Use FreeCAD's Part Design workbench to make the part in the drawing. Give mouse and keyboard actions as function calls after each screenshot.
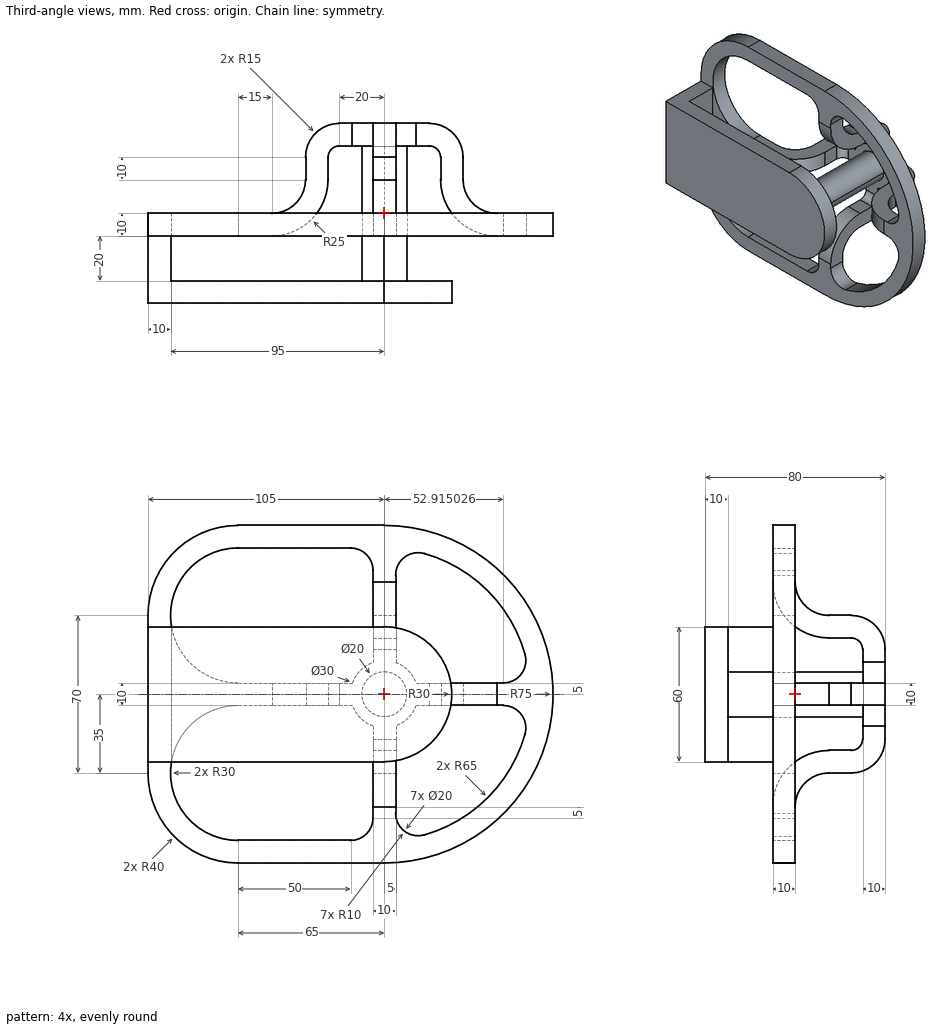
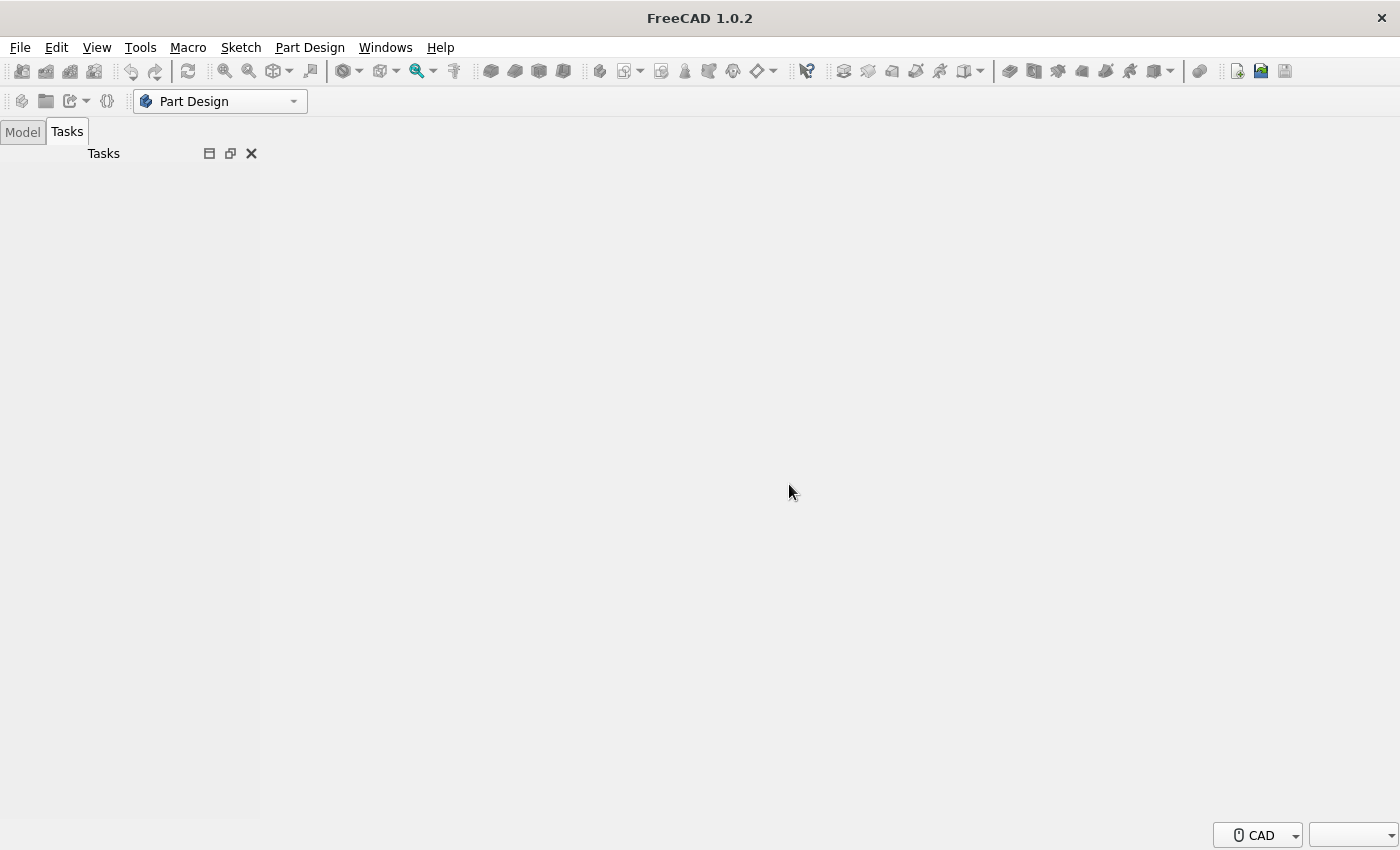
click(1238, 72)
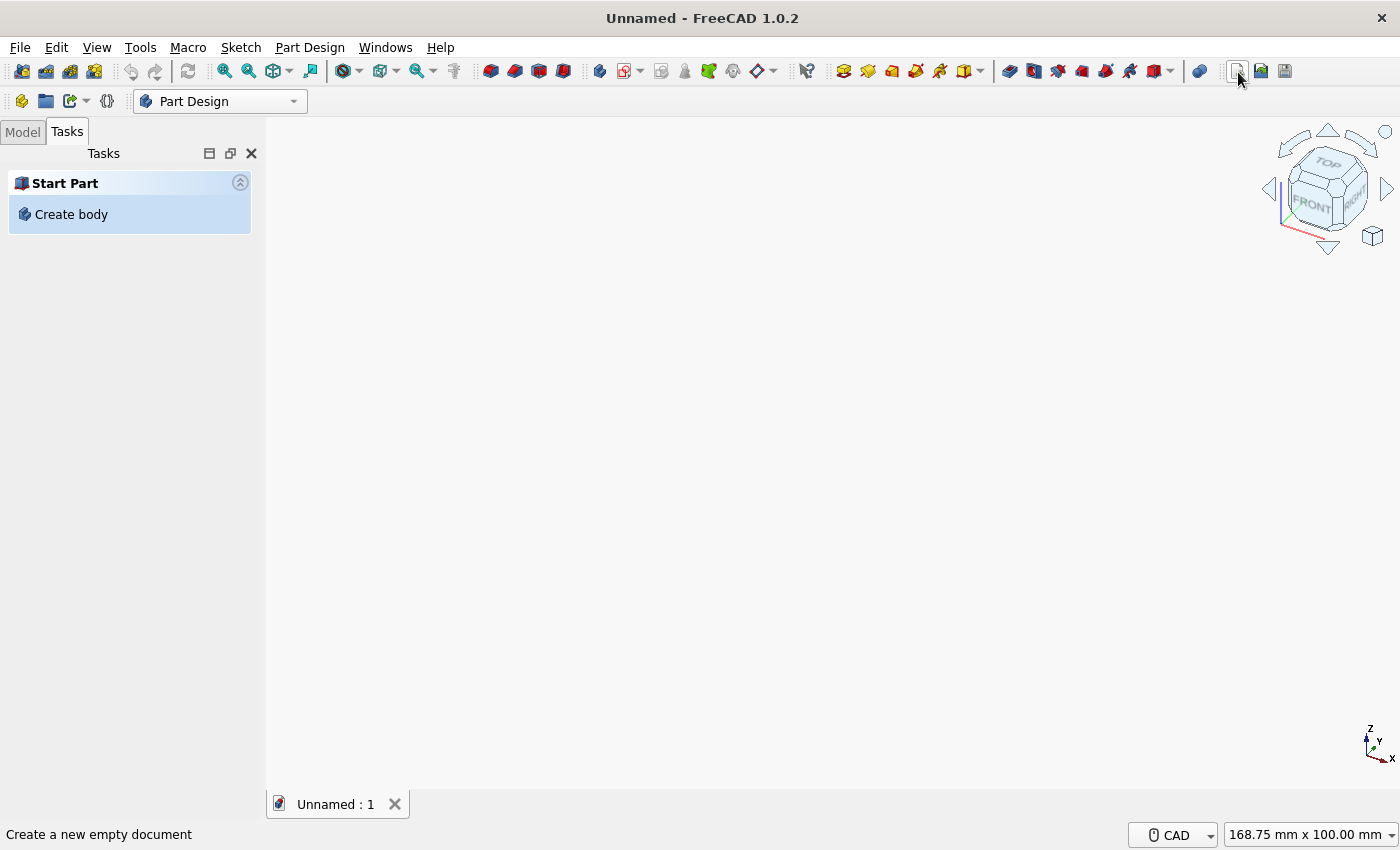
click(624, 72)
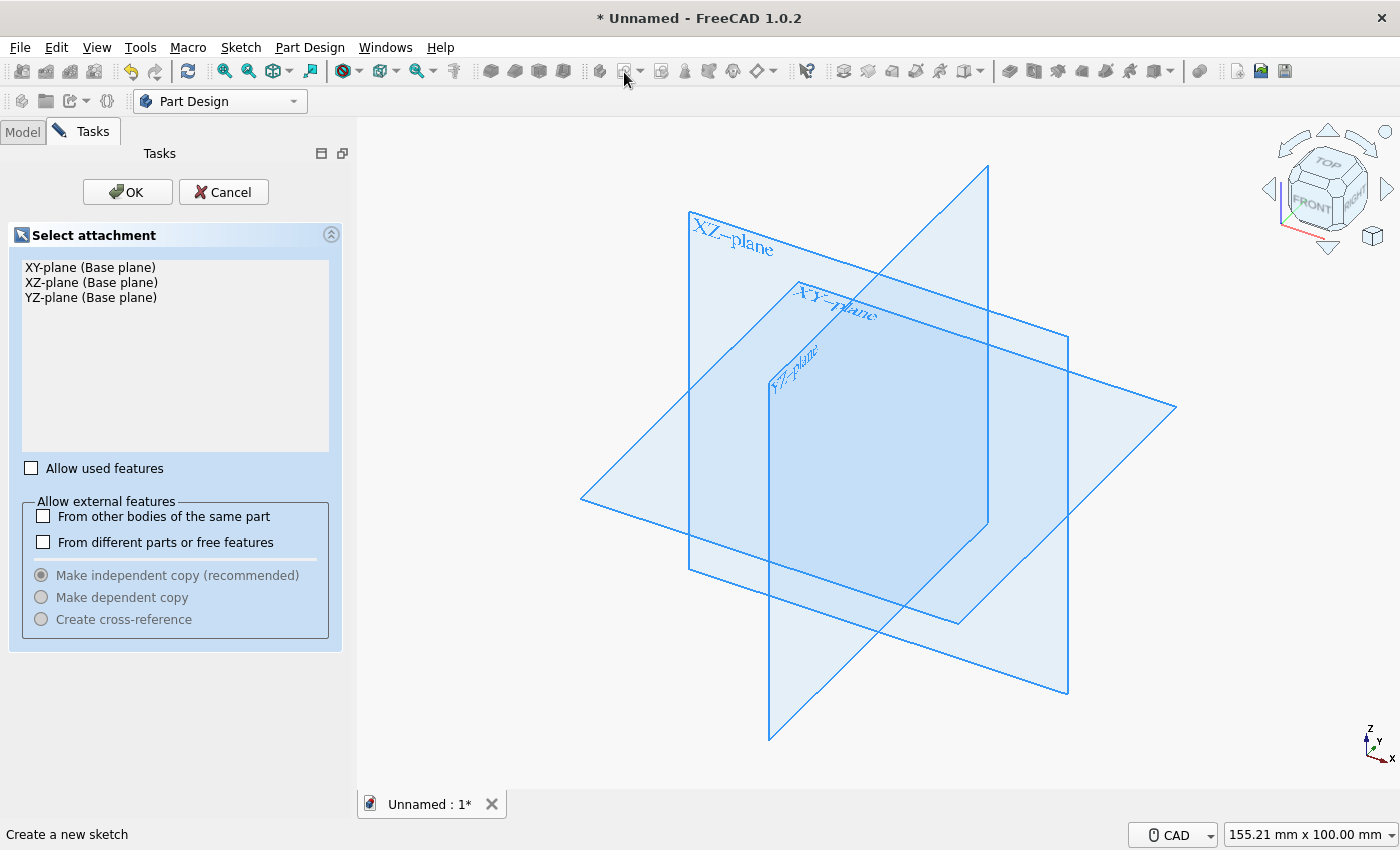
click(82, 282)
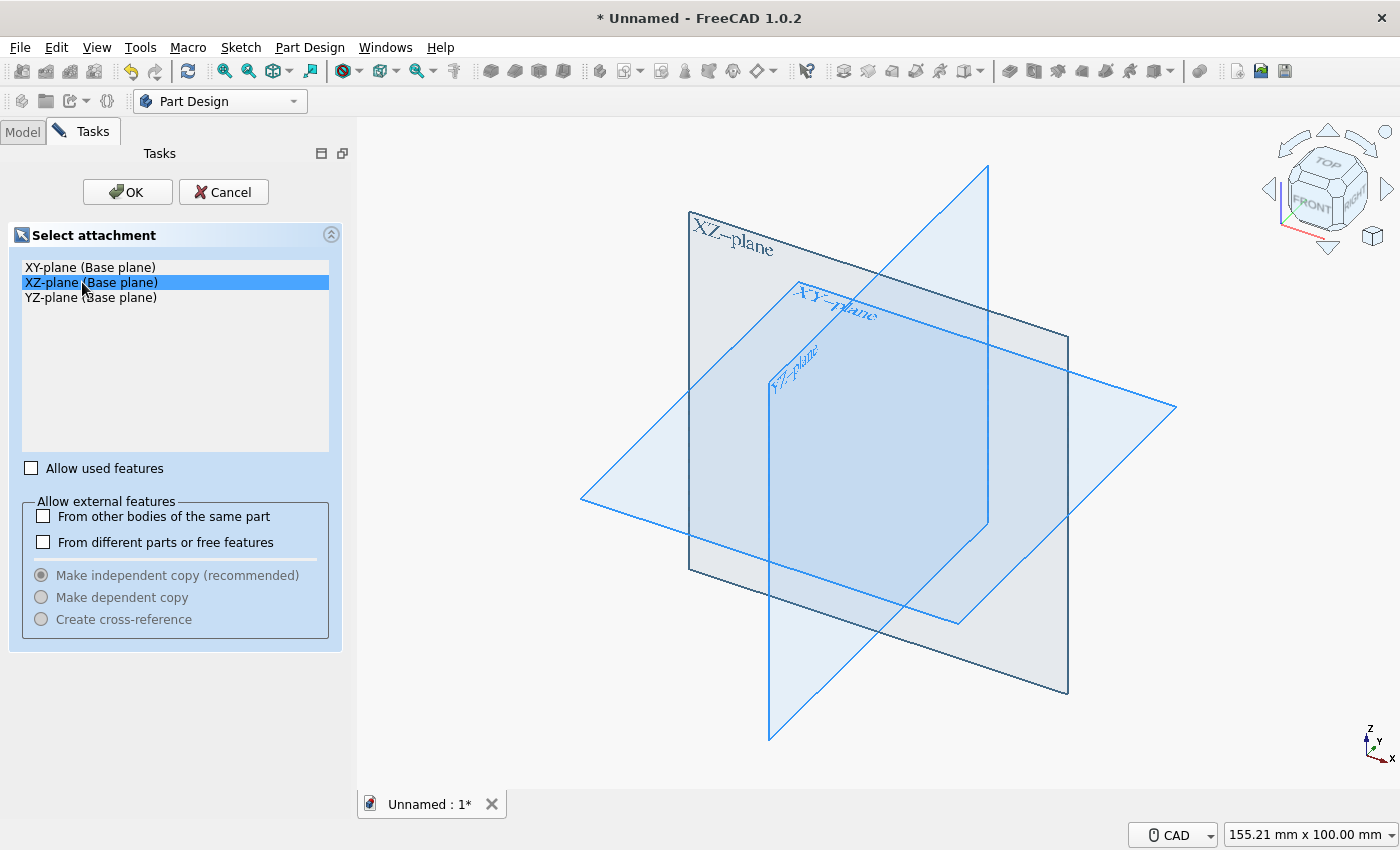
click(128, 192)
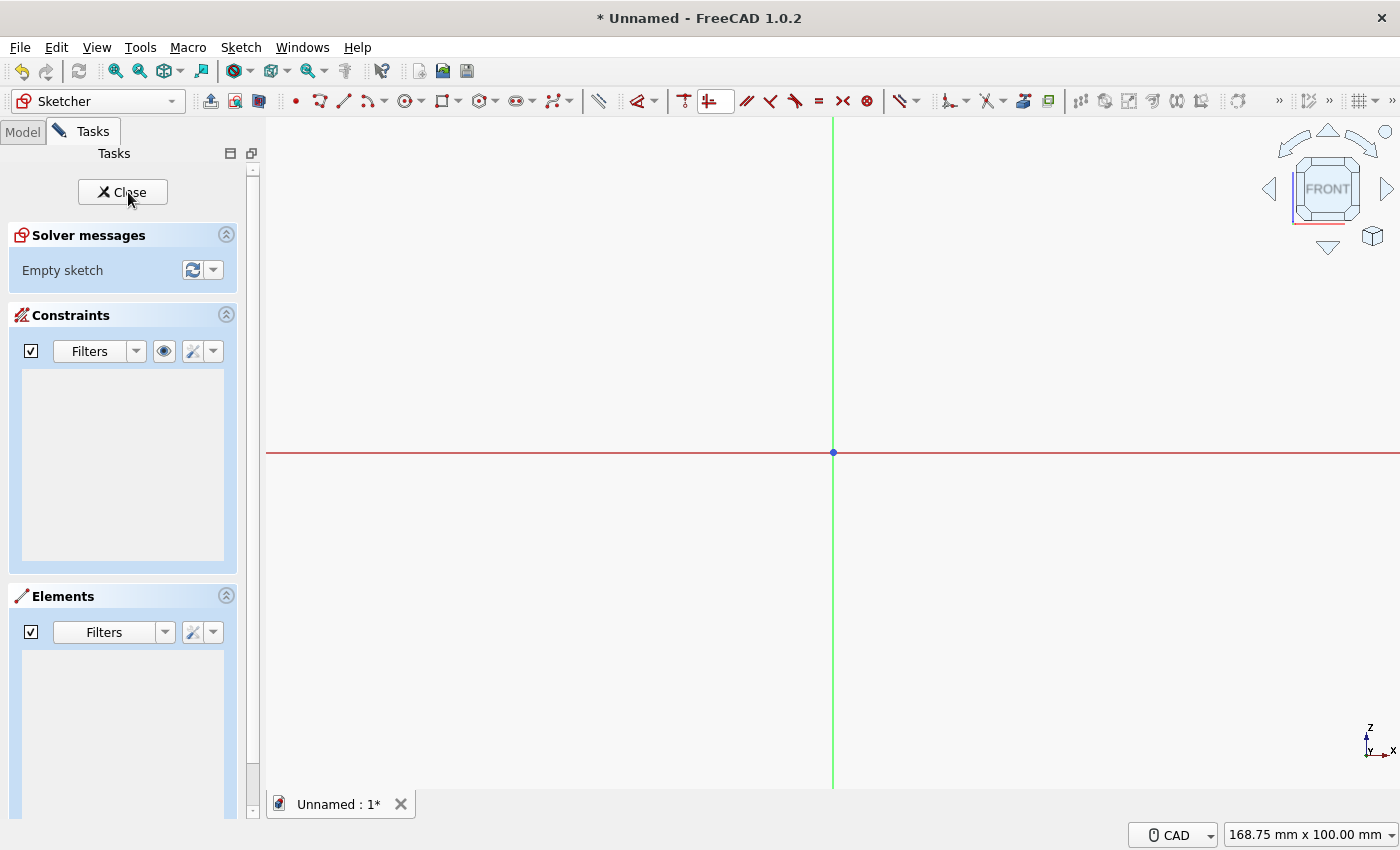
scroll(863, 453, up, 6)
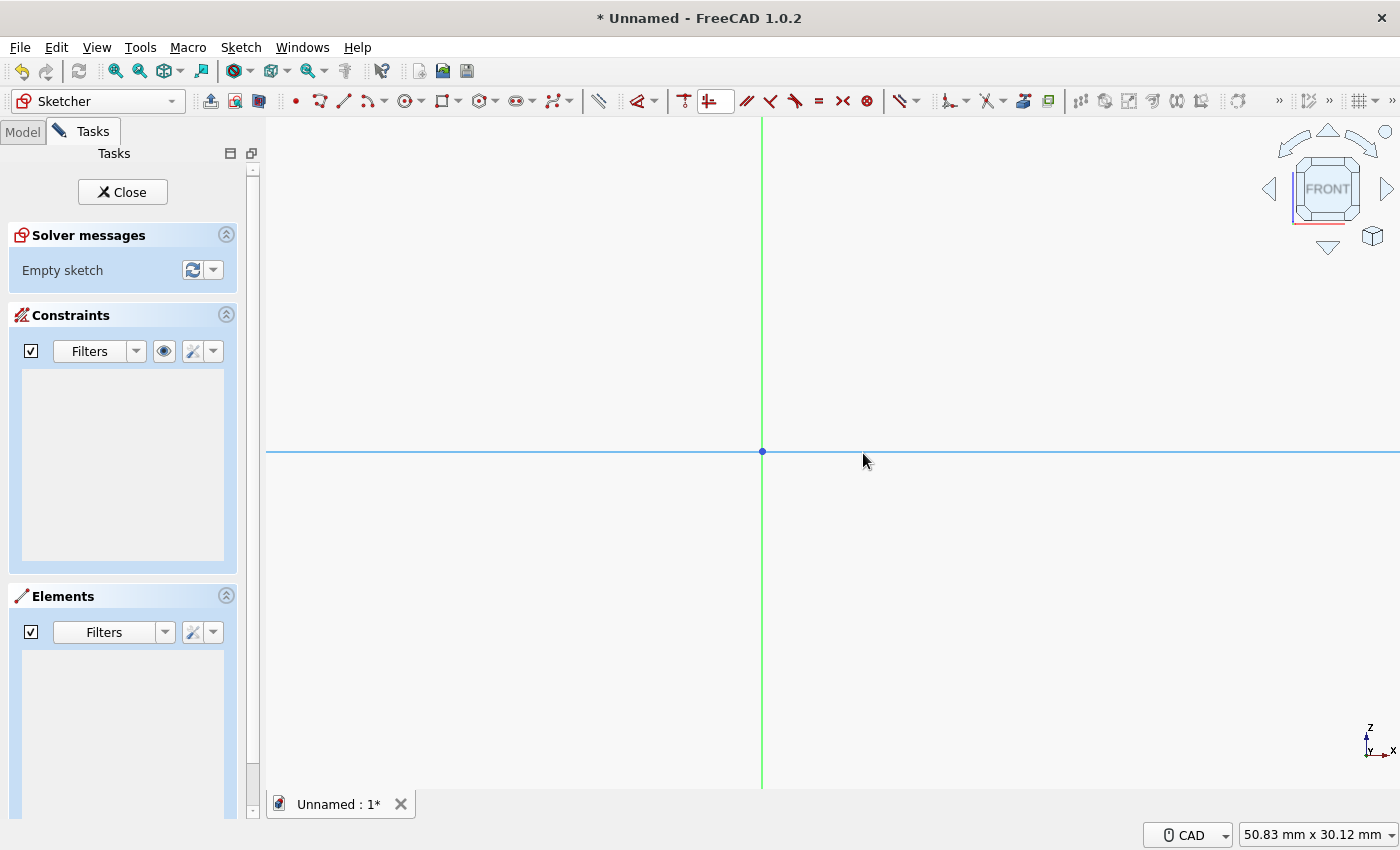
click(406, 102)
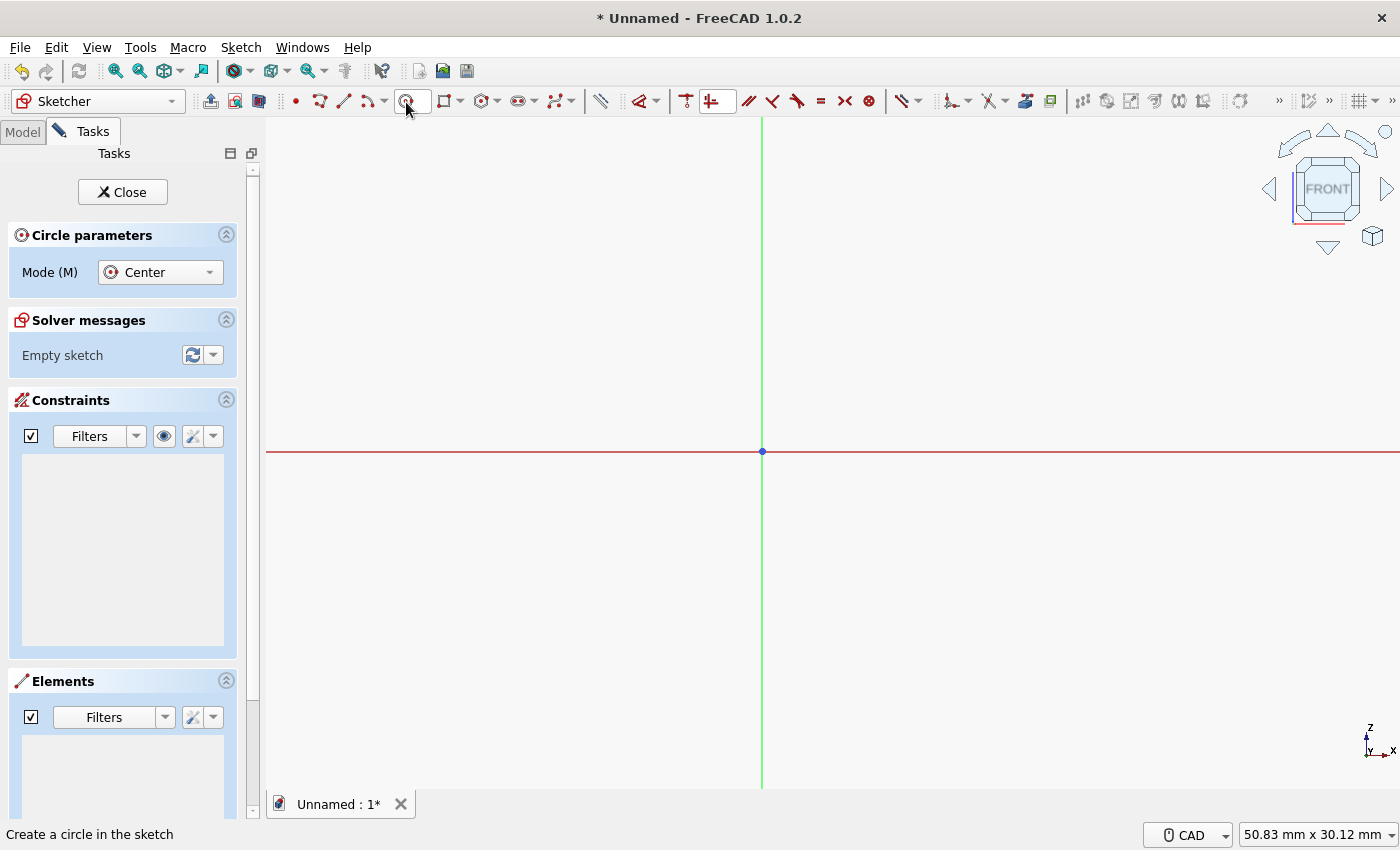
click(762, 452)
move(920, 294)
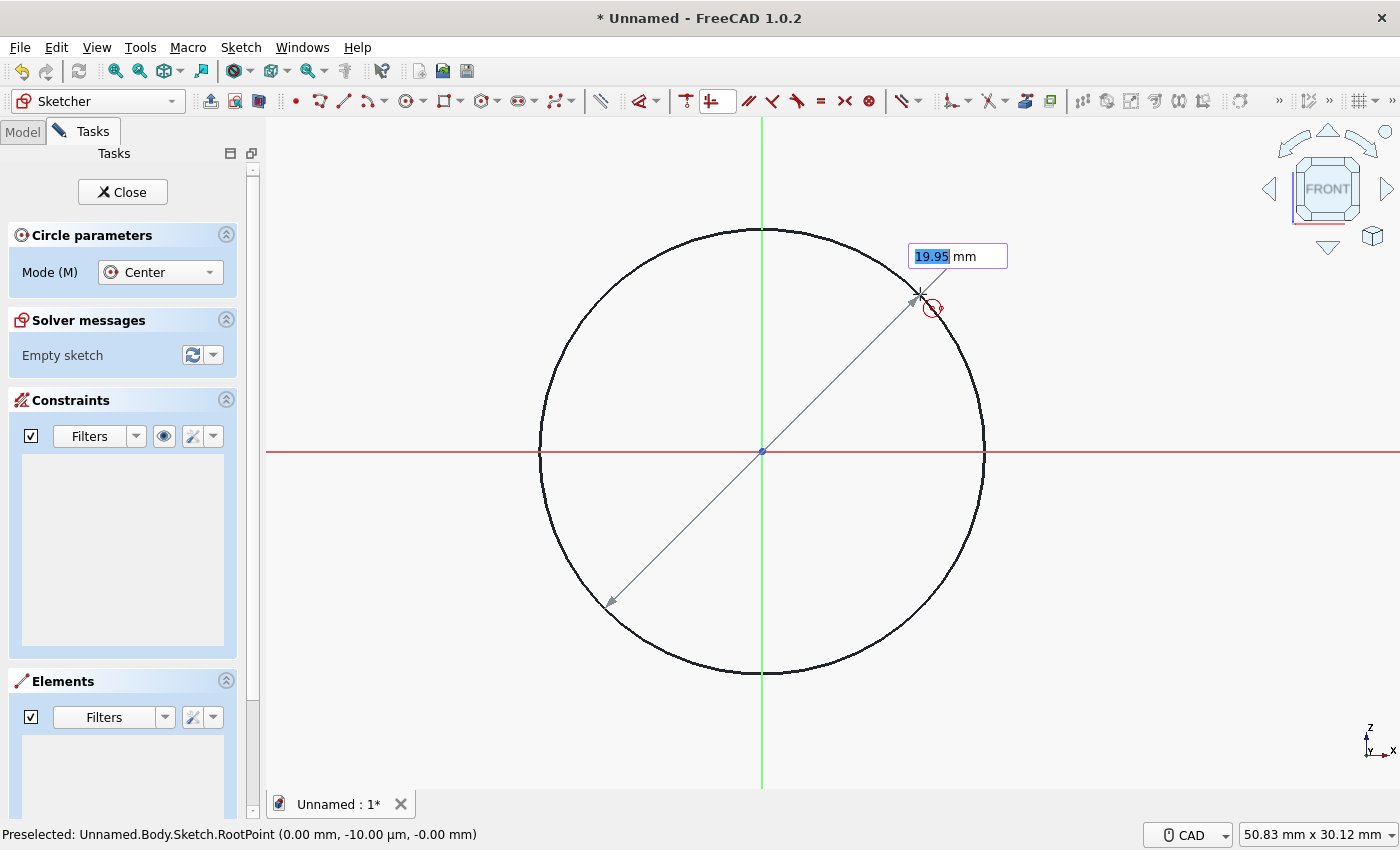
text(20)
key(Return)
key(Escape)